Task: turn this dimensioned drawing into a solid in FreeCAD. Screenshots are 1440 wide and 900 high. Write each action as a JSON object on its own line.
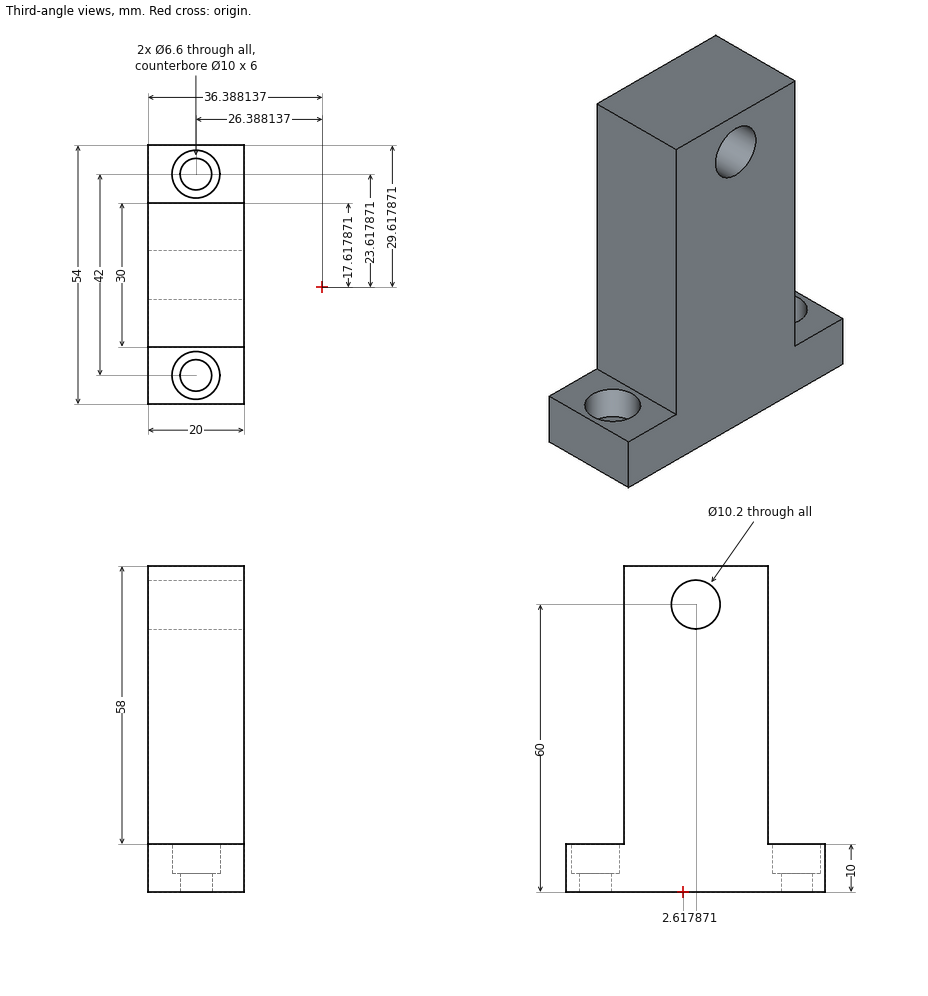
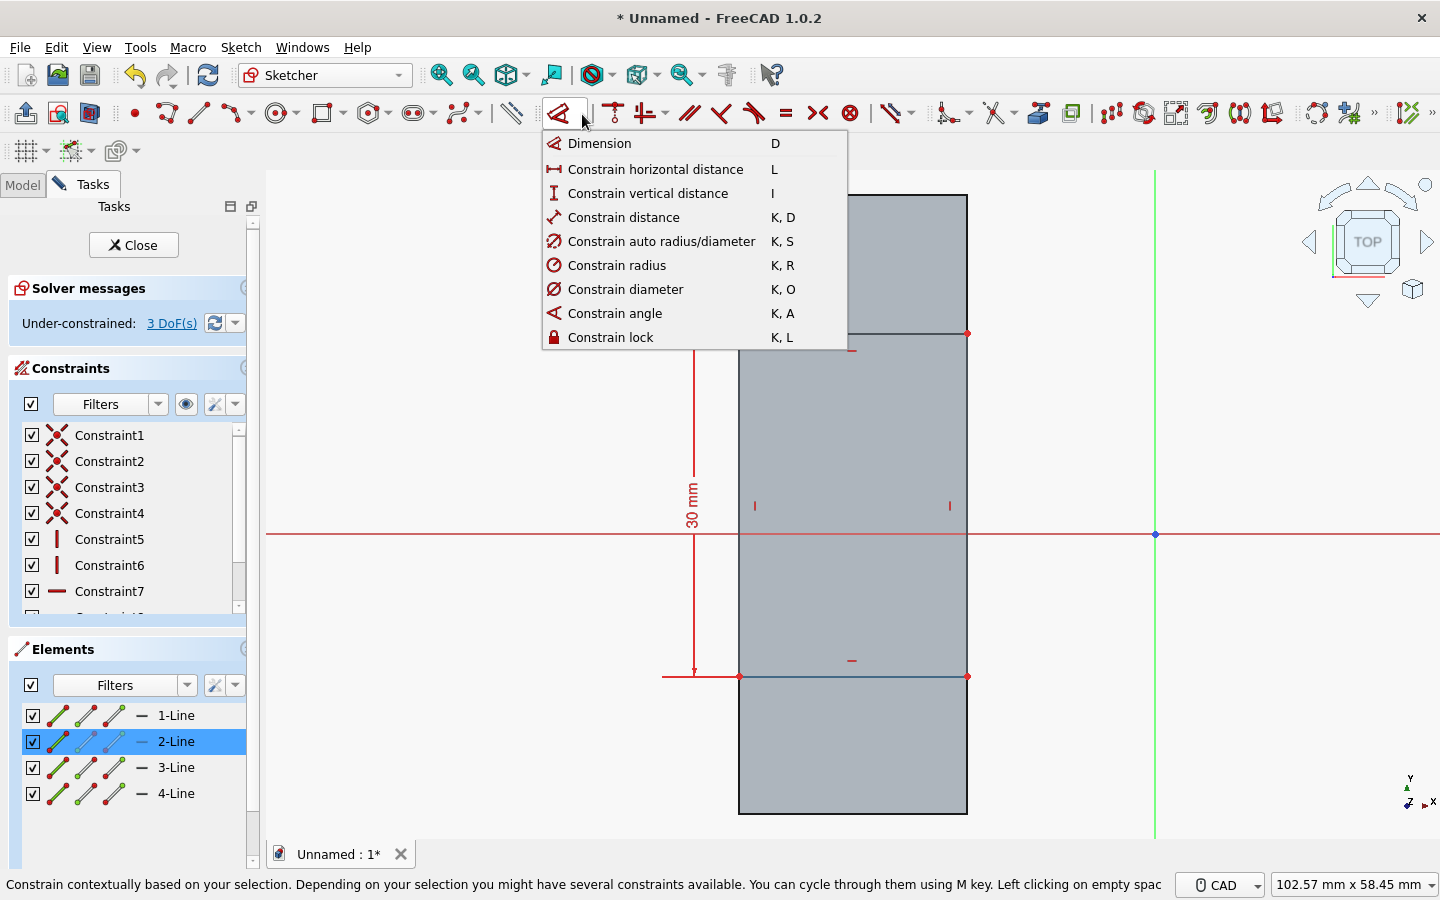
{"action": "left_click", "coordinate": [695, 169]}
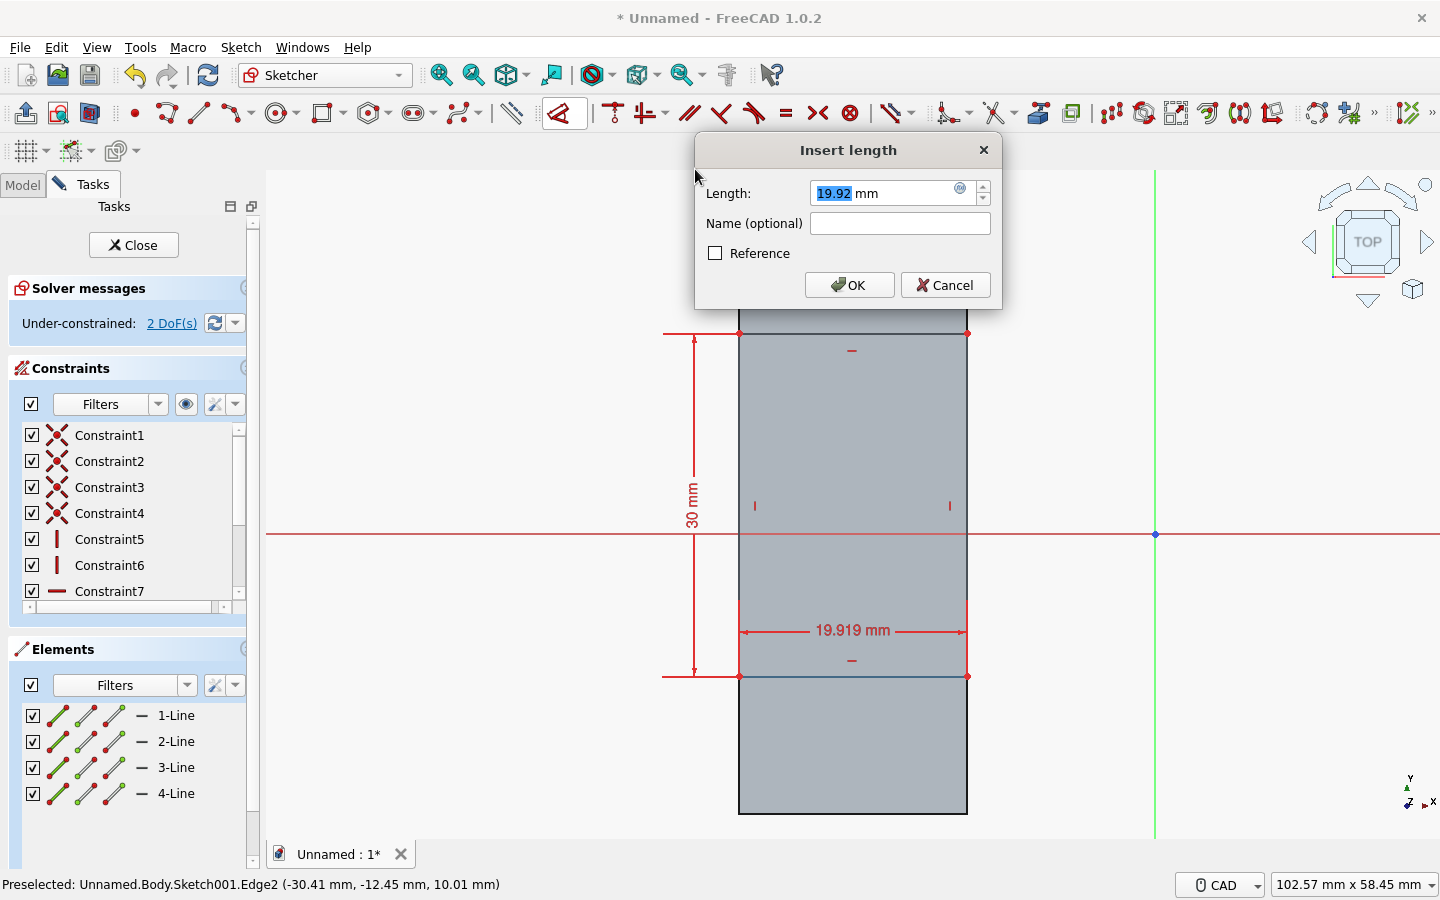
{"action": "type", "text": "20"}
{"action": "key", "text": "Return"}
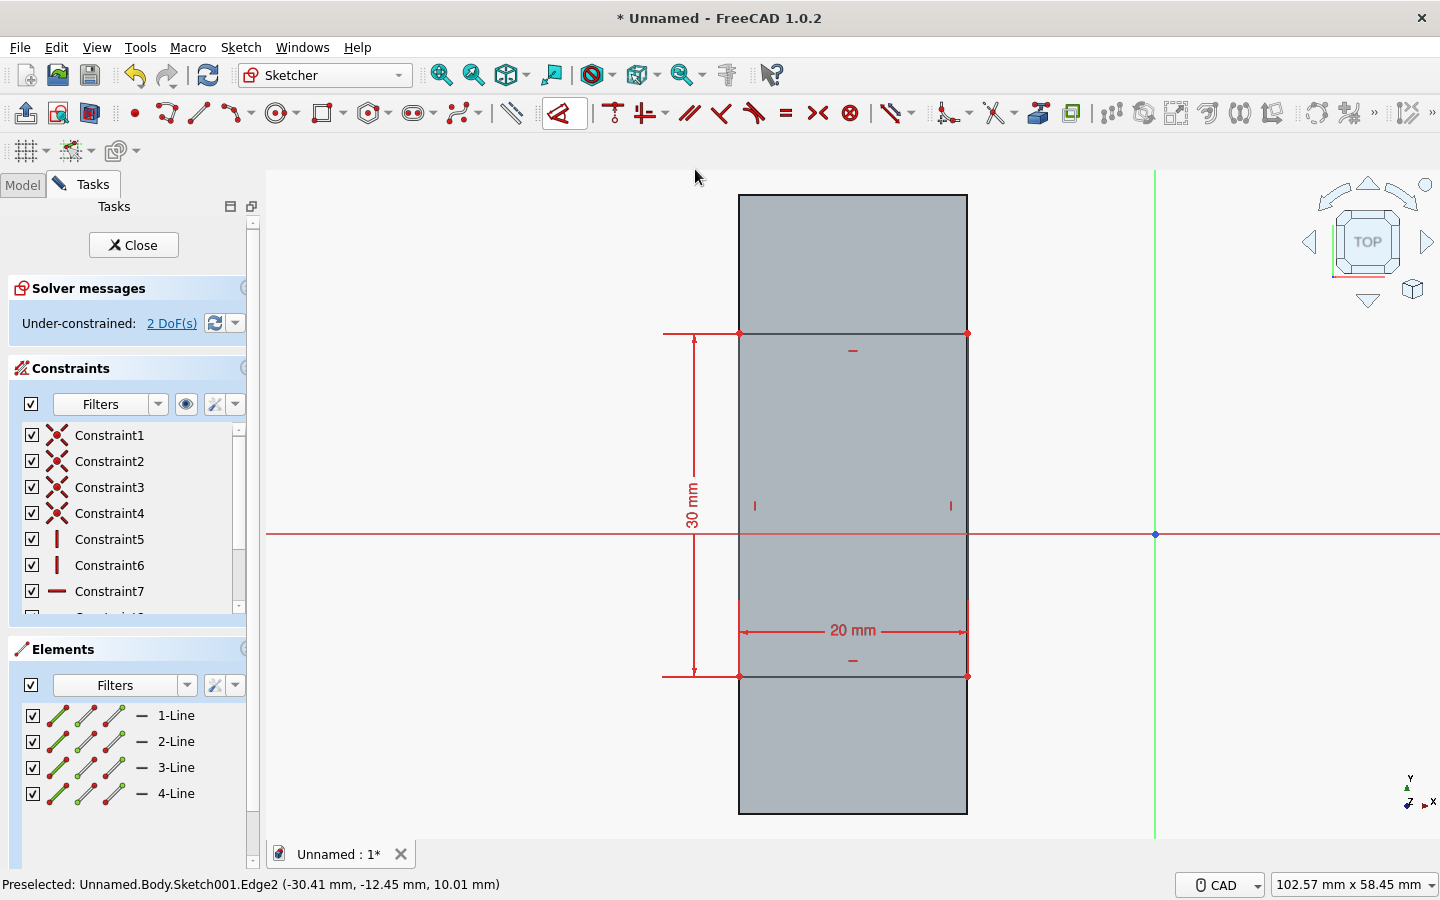
{"action": "left_click", "coordinate": [739, 334]}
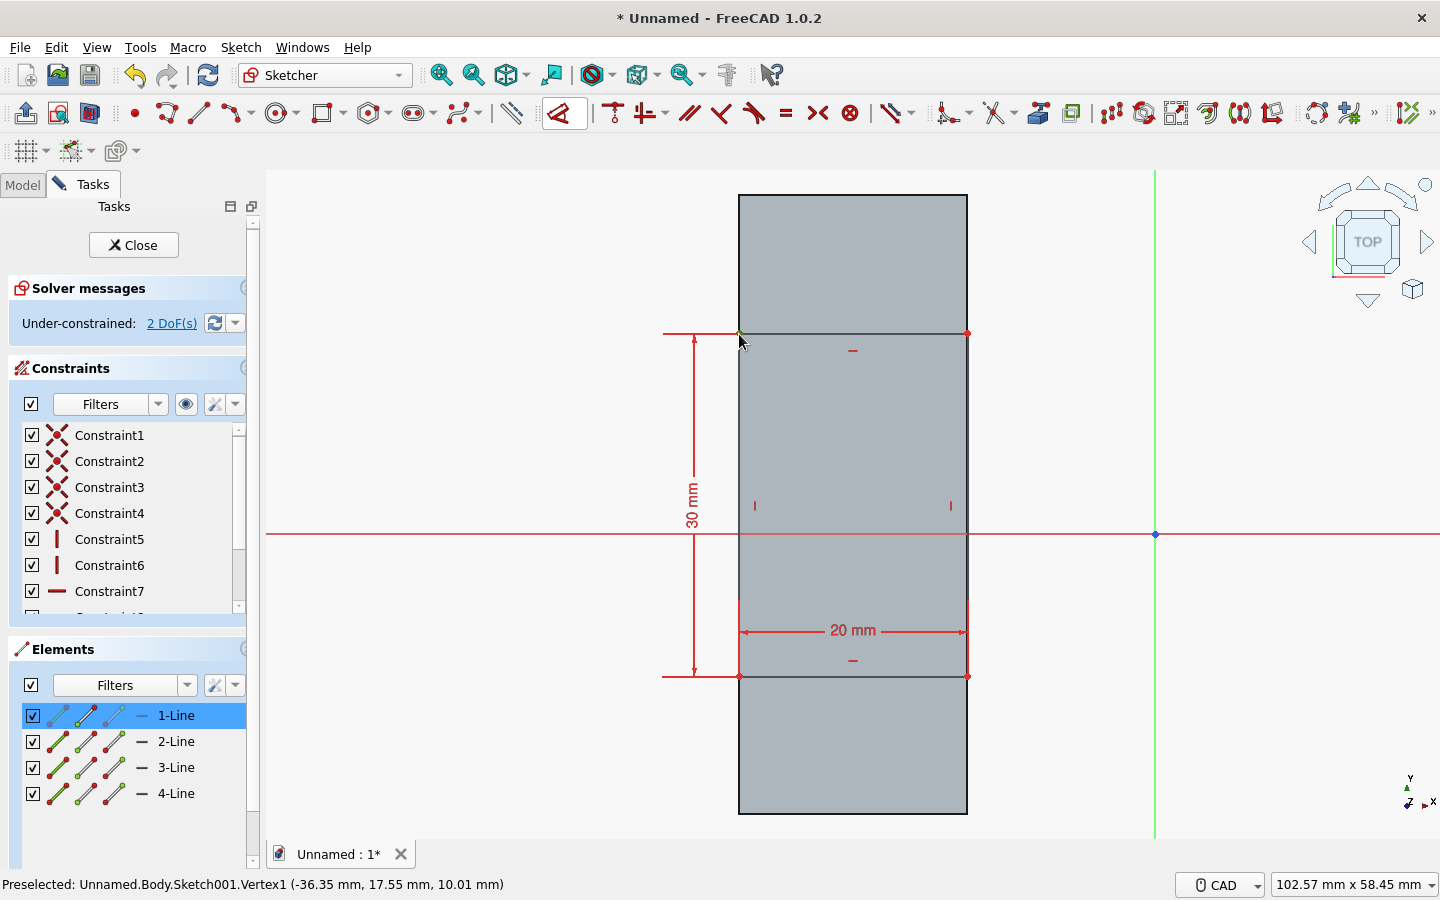
{"action": "key", "text": "l"}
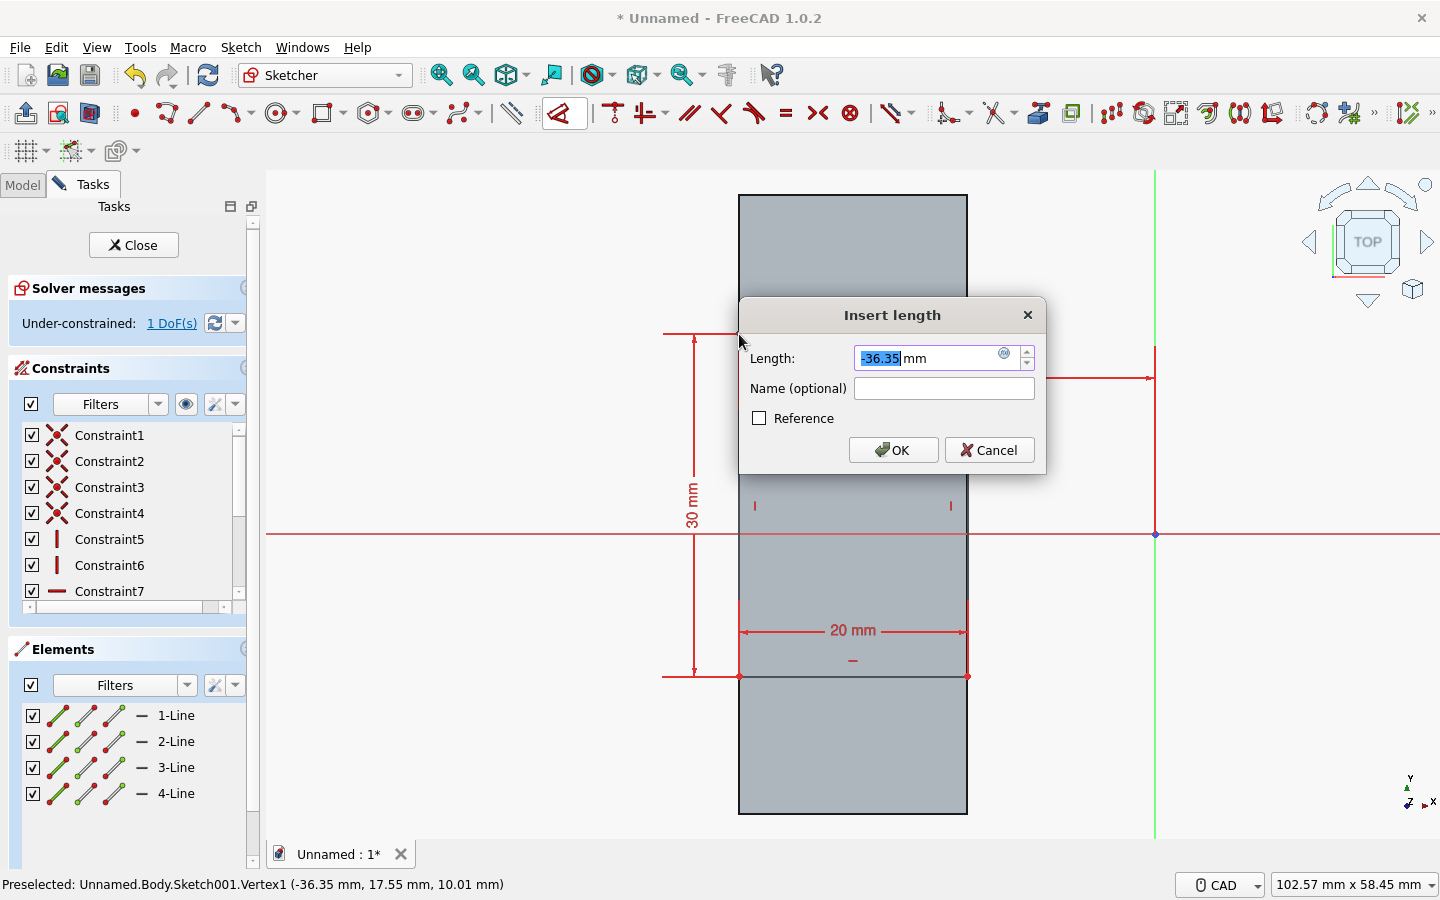
{"action": "type", "text": "-36.388137"}
{"action": "key", "text": "Return"}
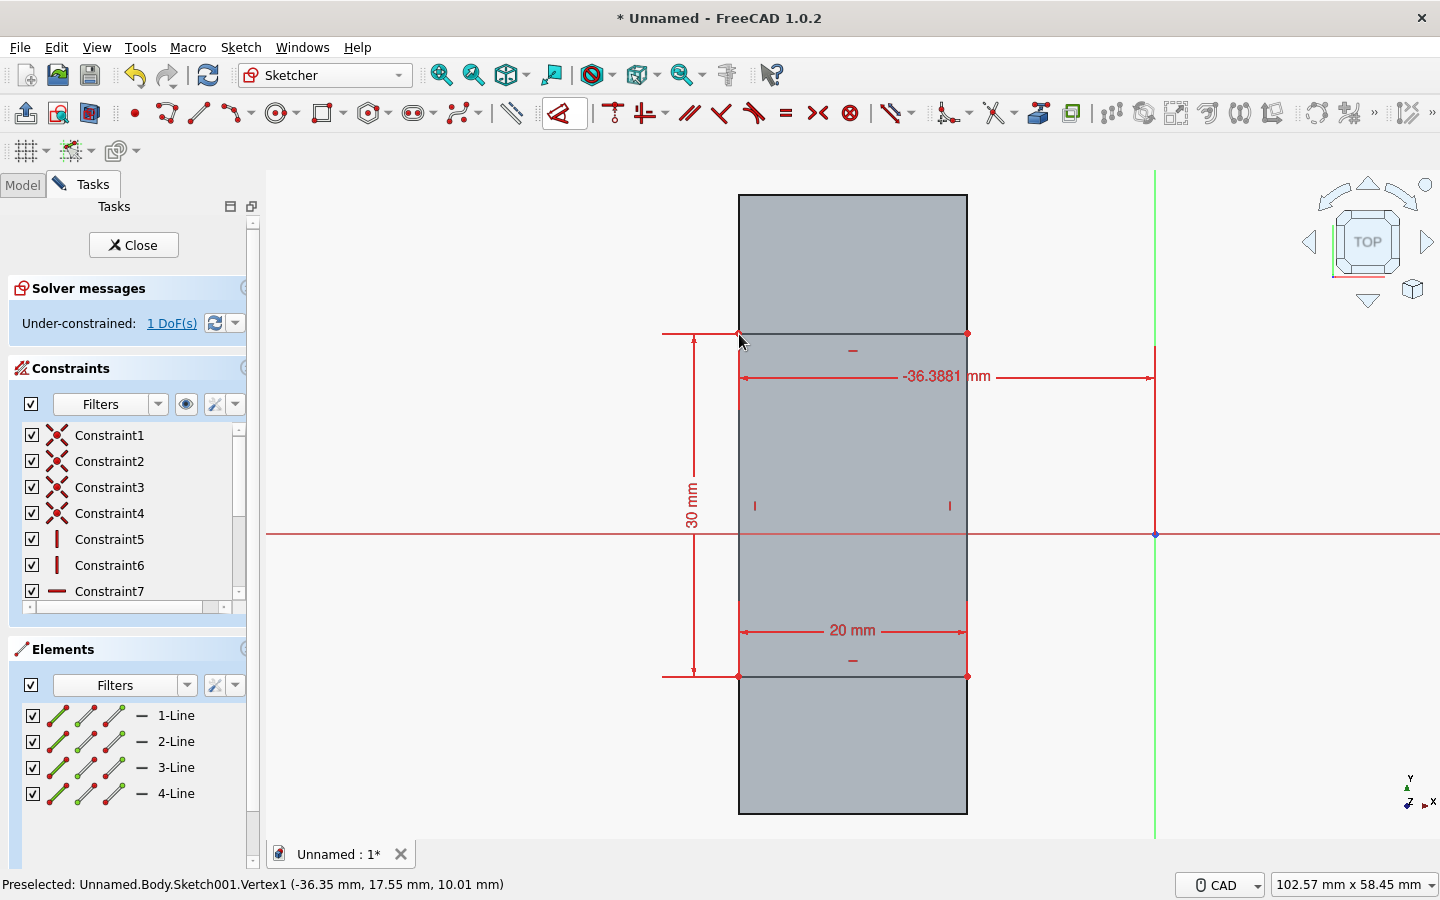
{"action": "left_click", "coordinate": [739, 334]}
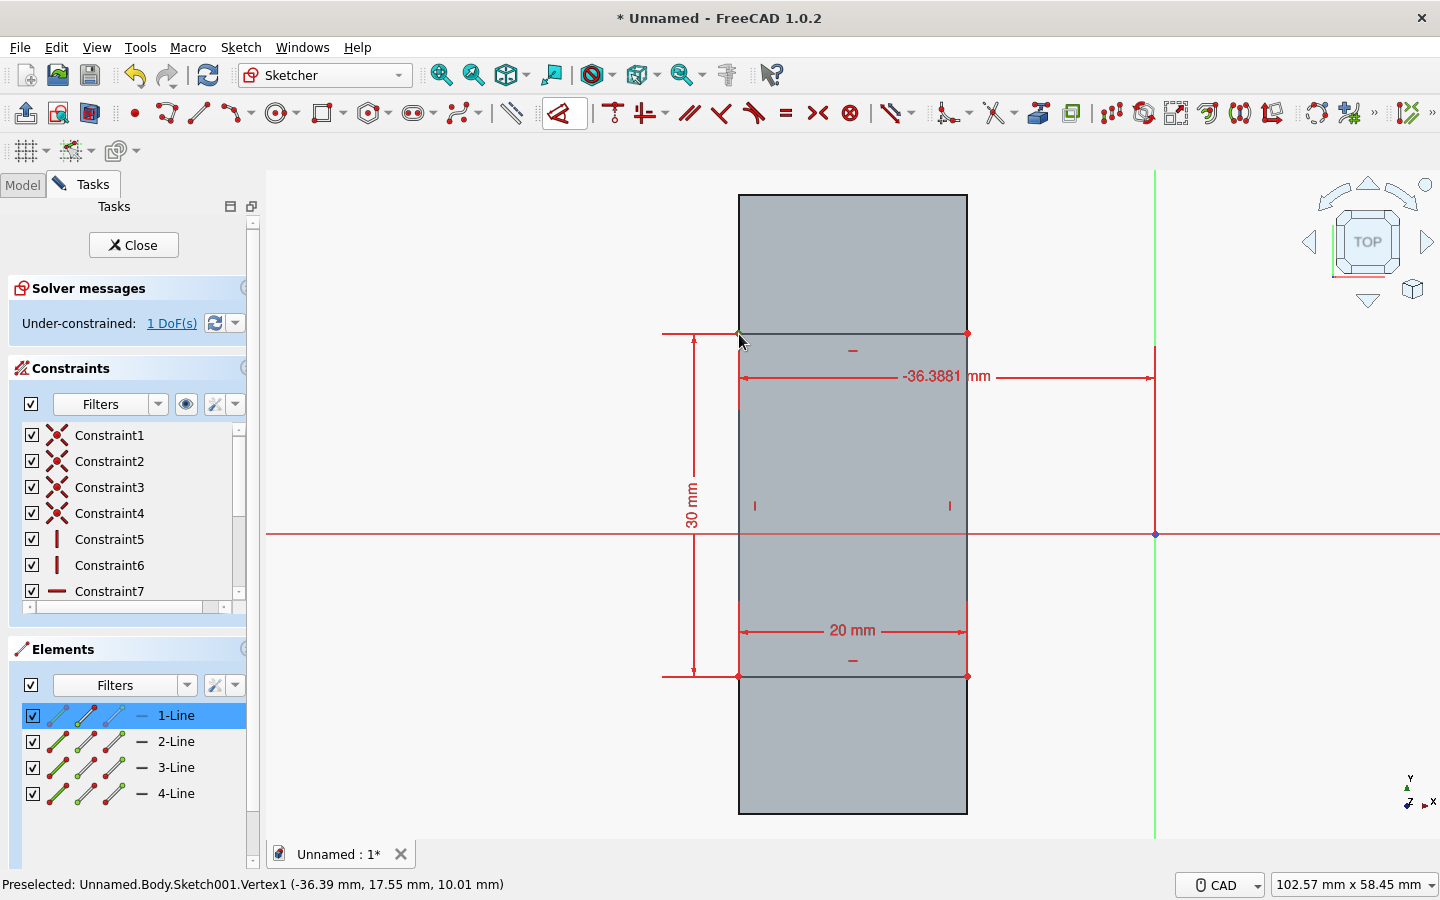
{"action": "key", "text": "i"}